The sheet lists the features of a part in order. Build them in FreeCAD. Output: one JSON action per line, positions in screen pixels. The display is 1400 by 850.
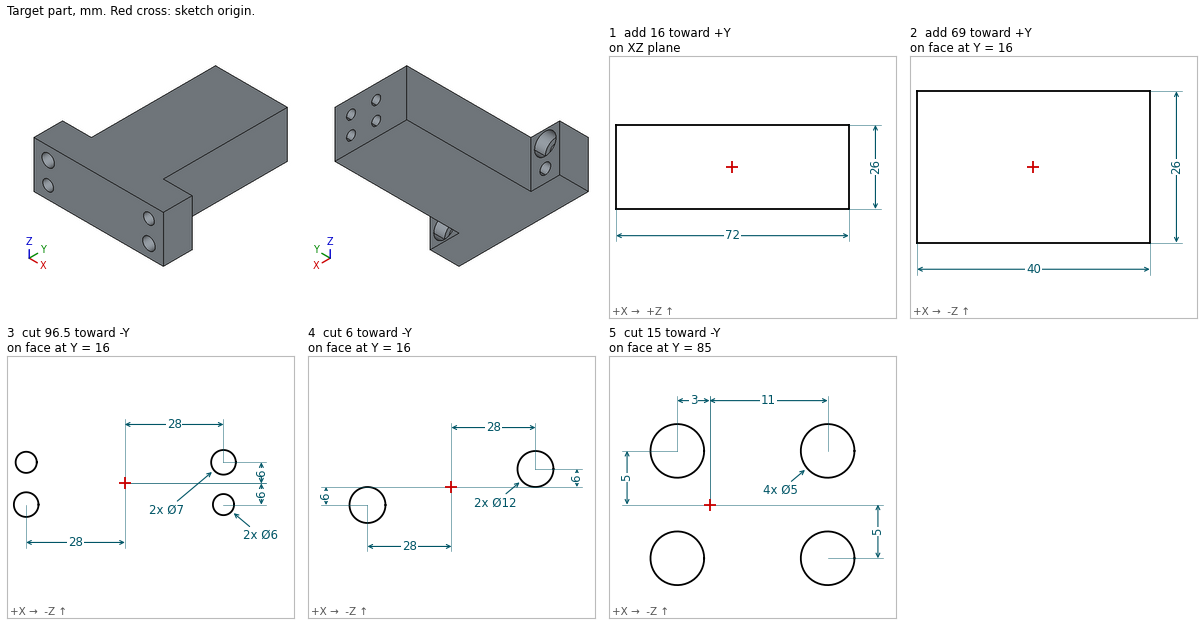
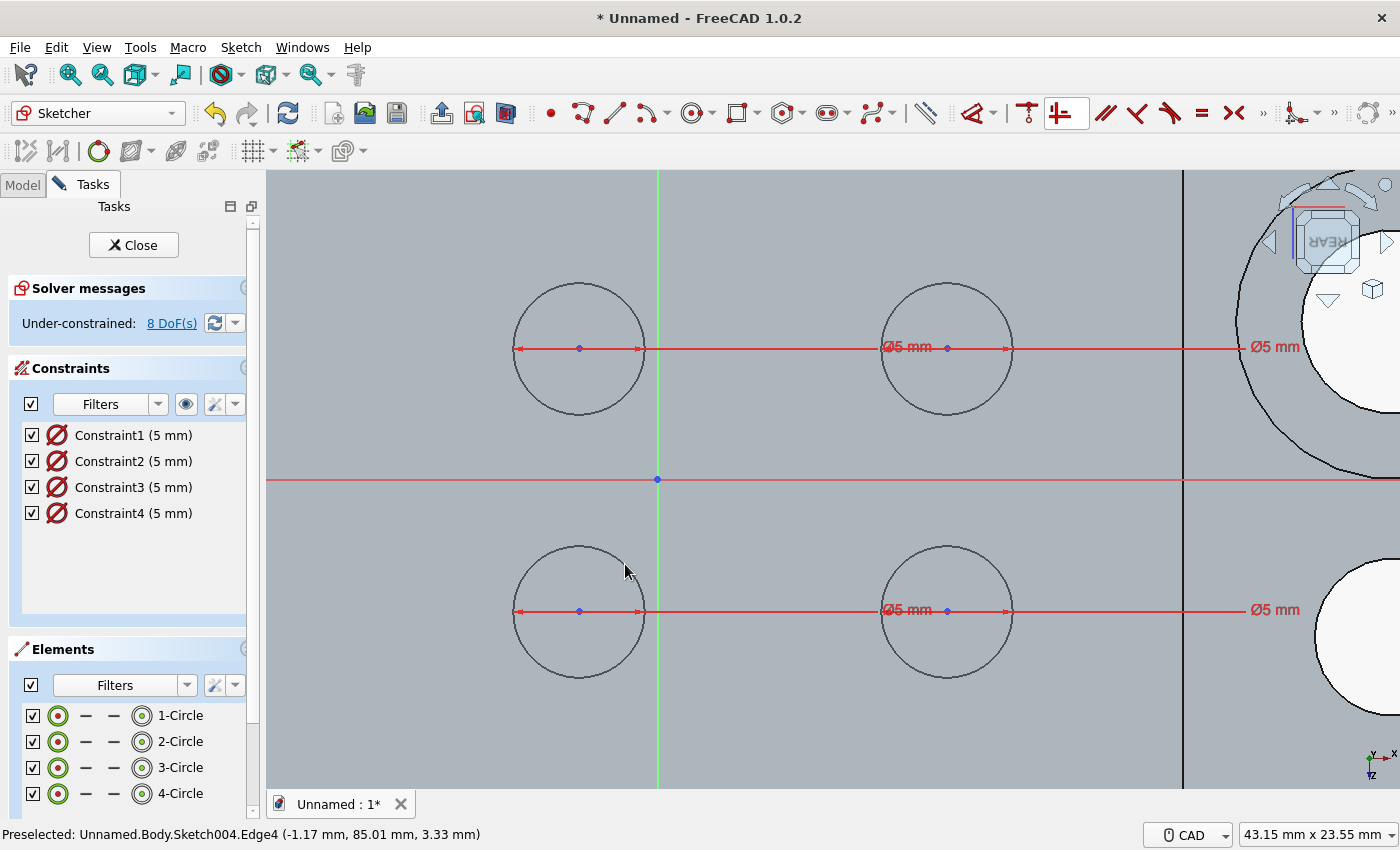
{"action": "left_click", "coordinate": [579, 349]}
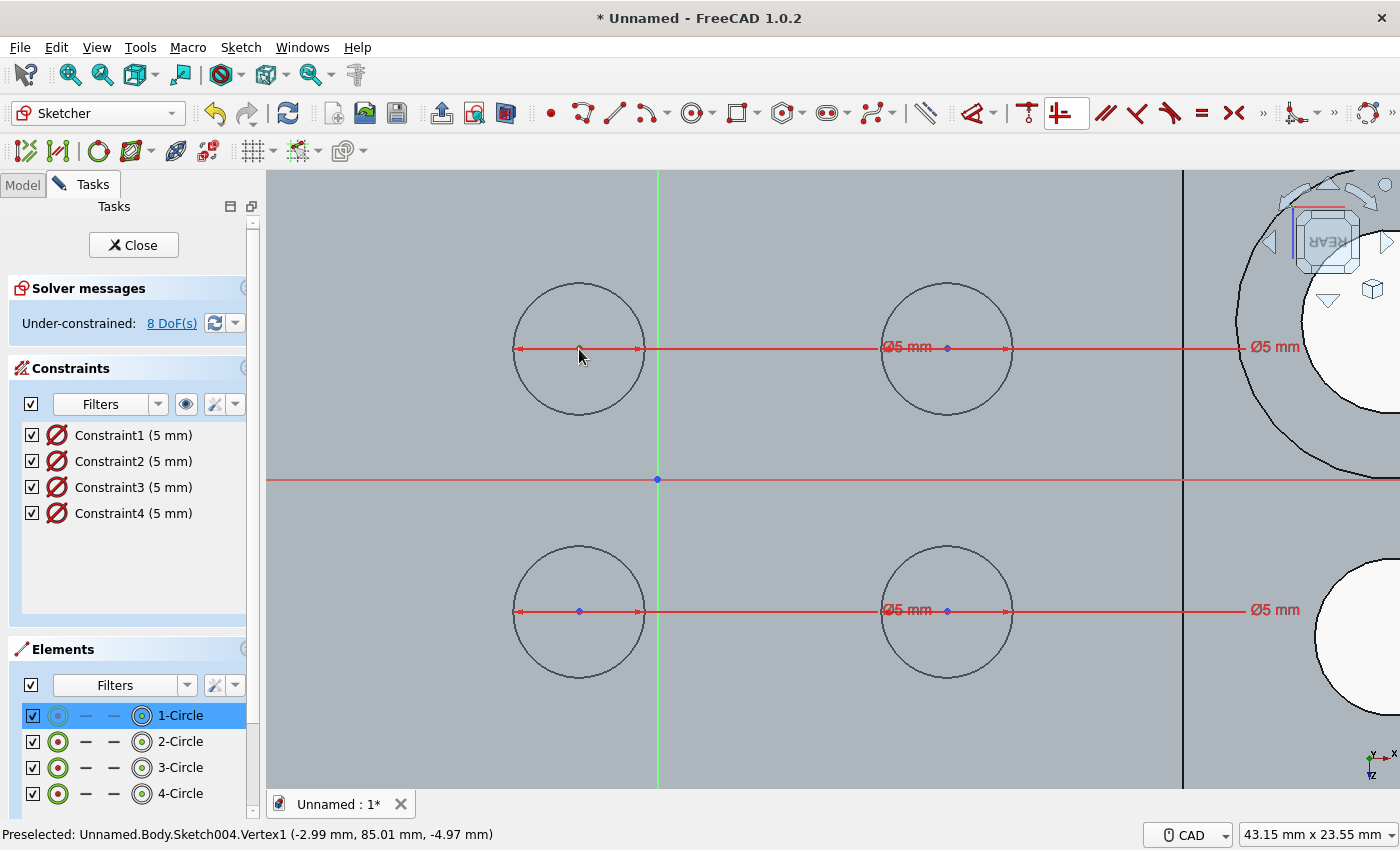
{"action": "left_click", "coordinate": [947, 349]}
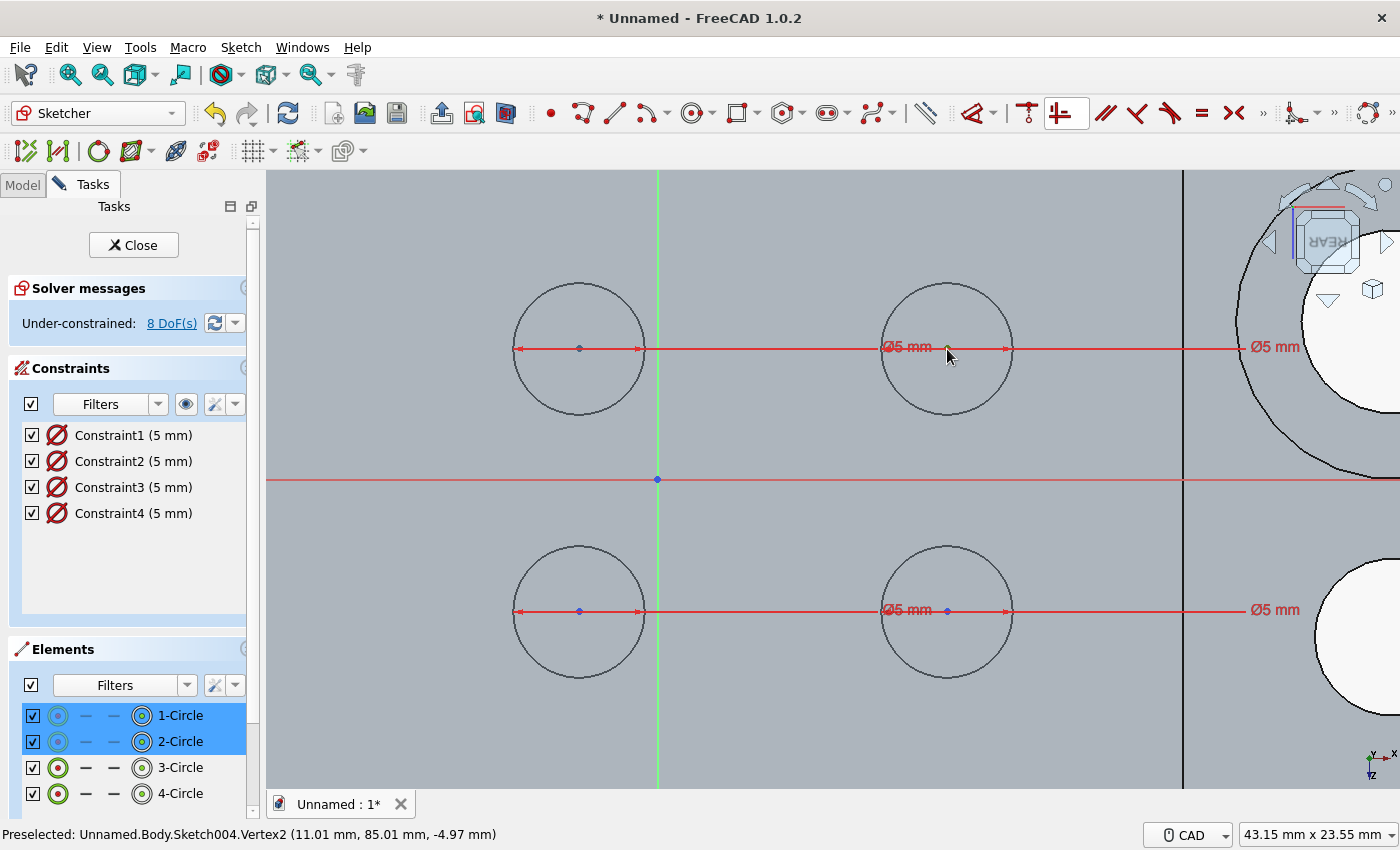
{"action": "key", "text": "h"}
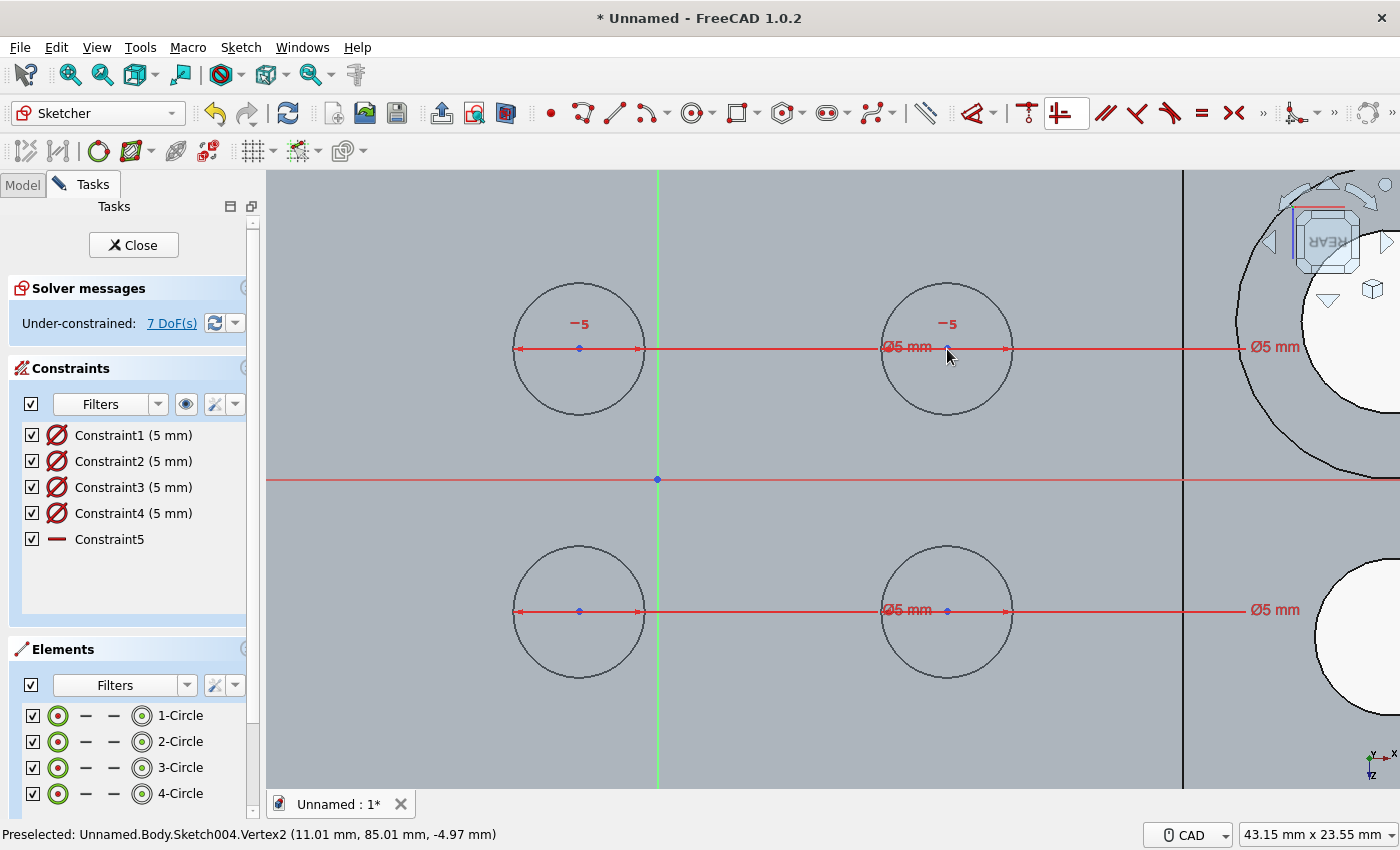
{"action": "left_click", "coordinate": [947, 349]}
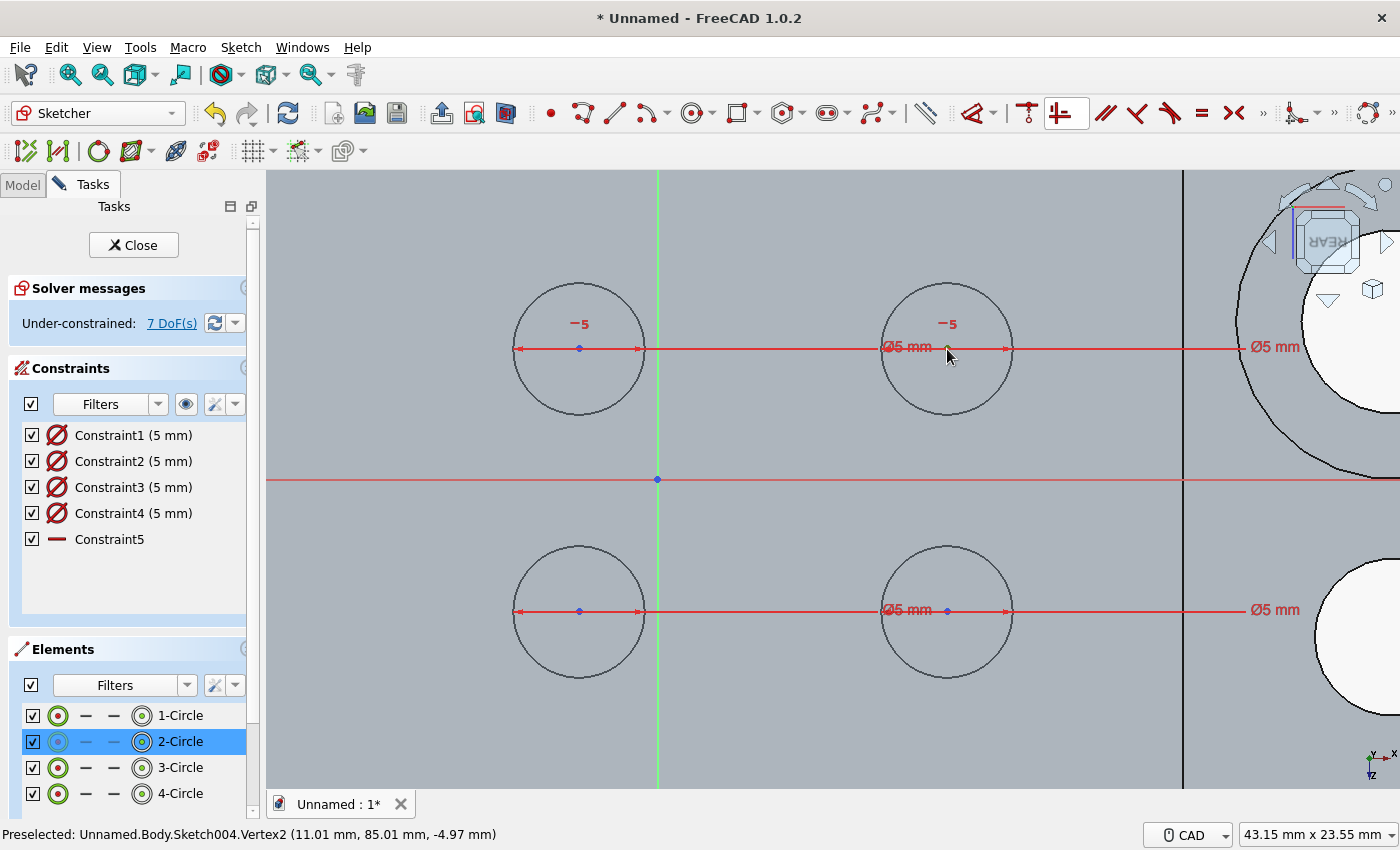
{"action": "left_click", "coordinate": [947, 612]}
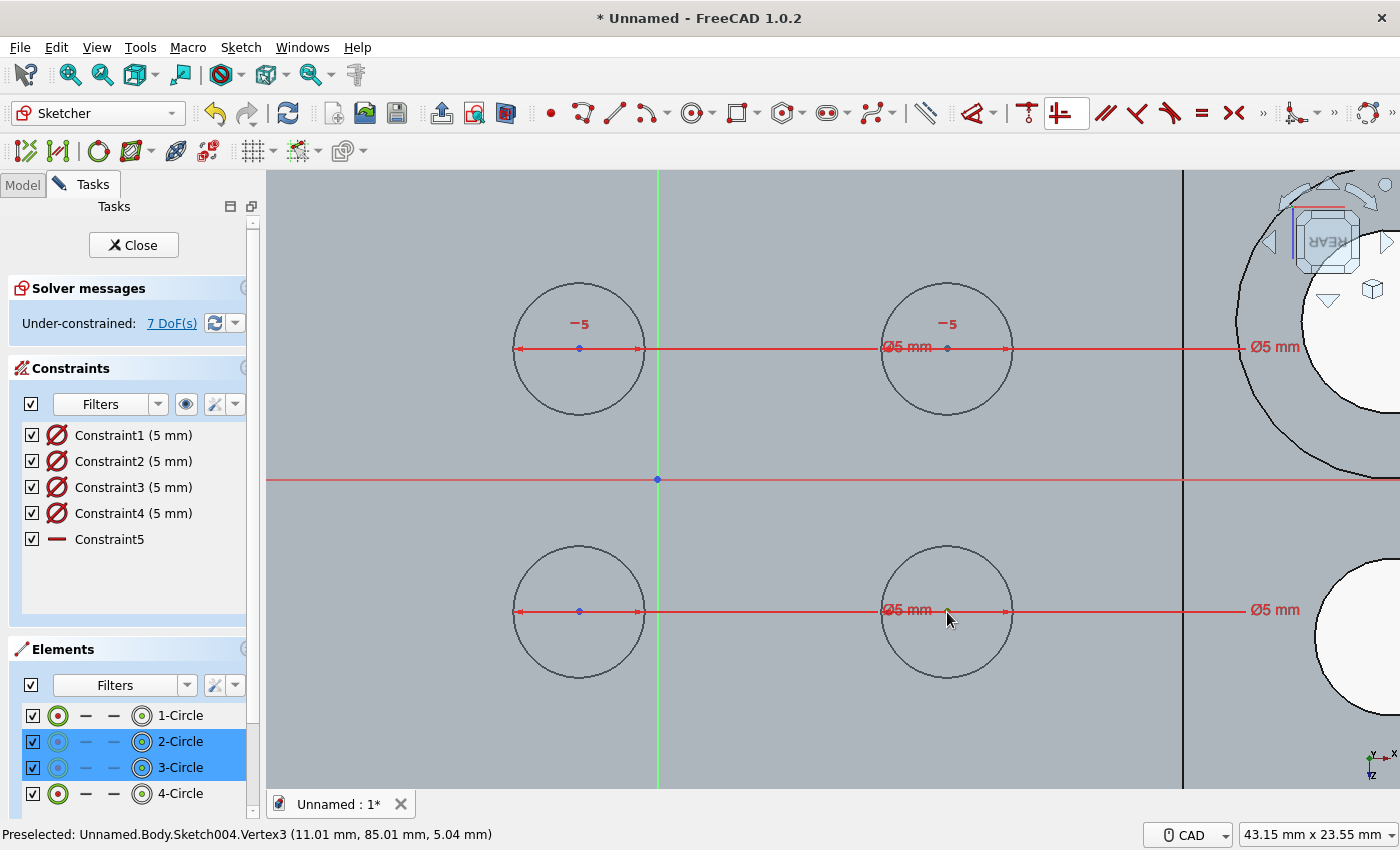
{"action": "key", "text": "v"}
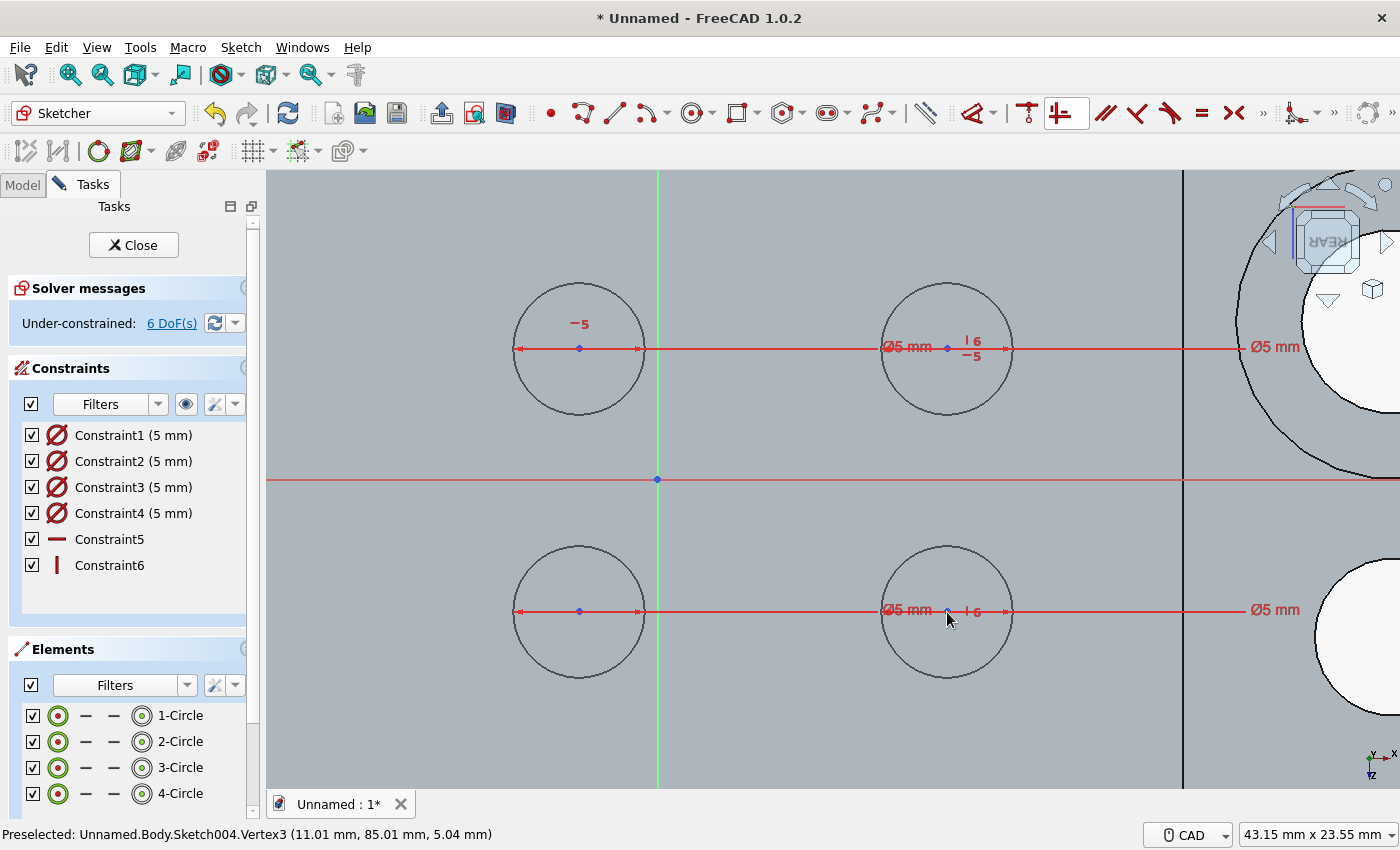
{"action": "left_click", "coordinate": [579, 349]}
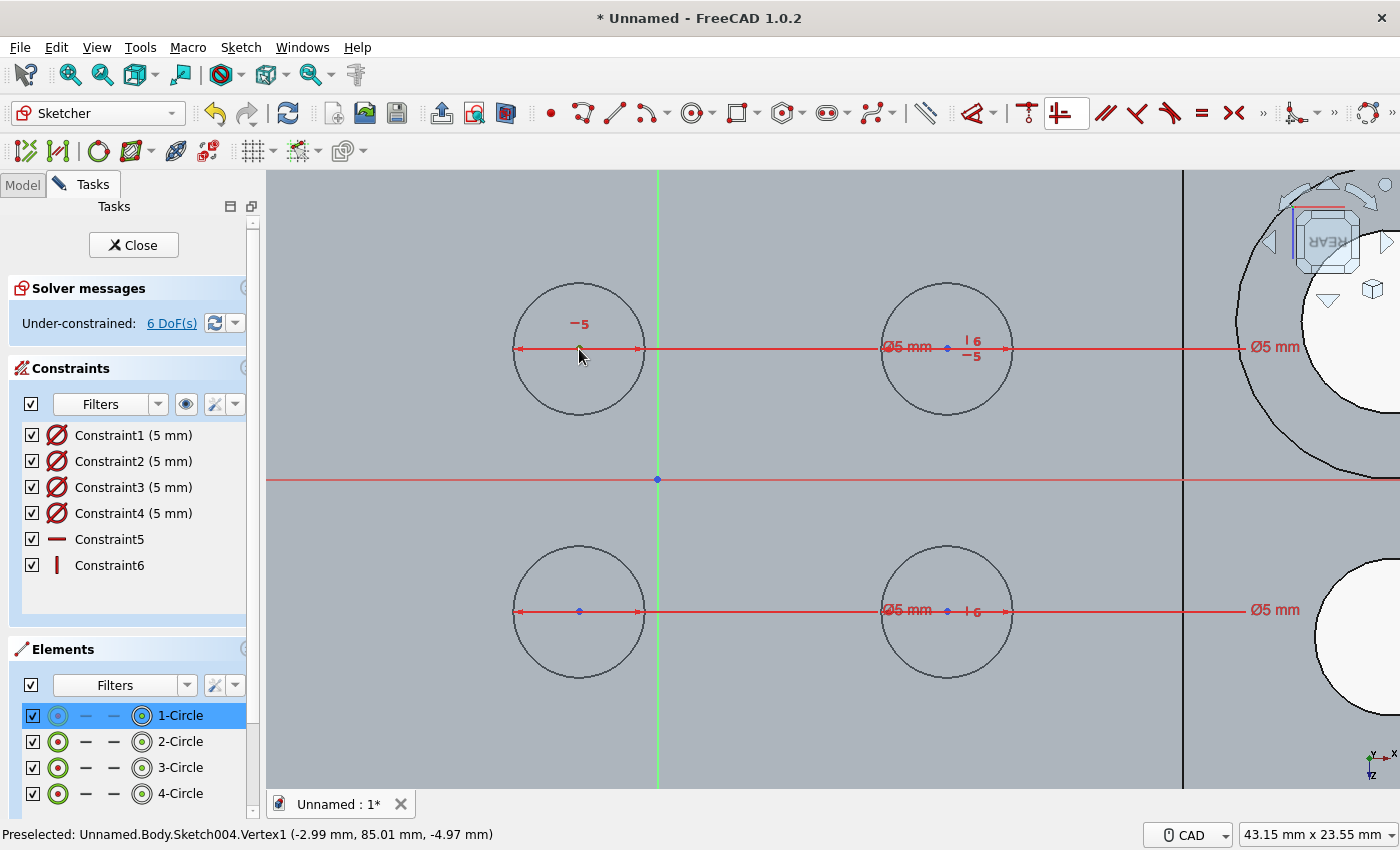
{"action": "left_click", "coordinate": [579, 612]}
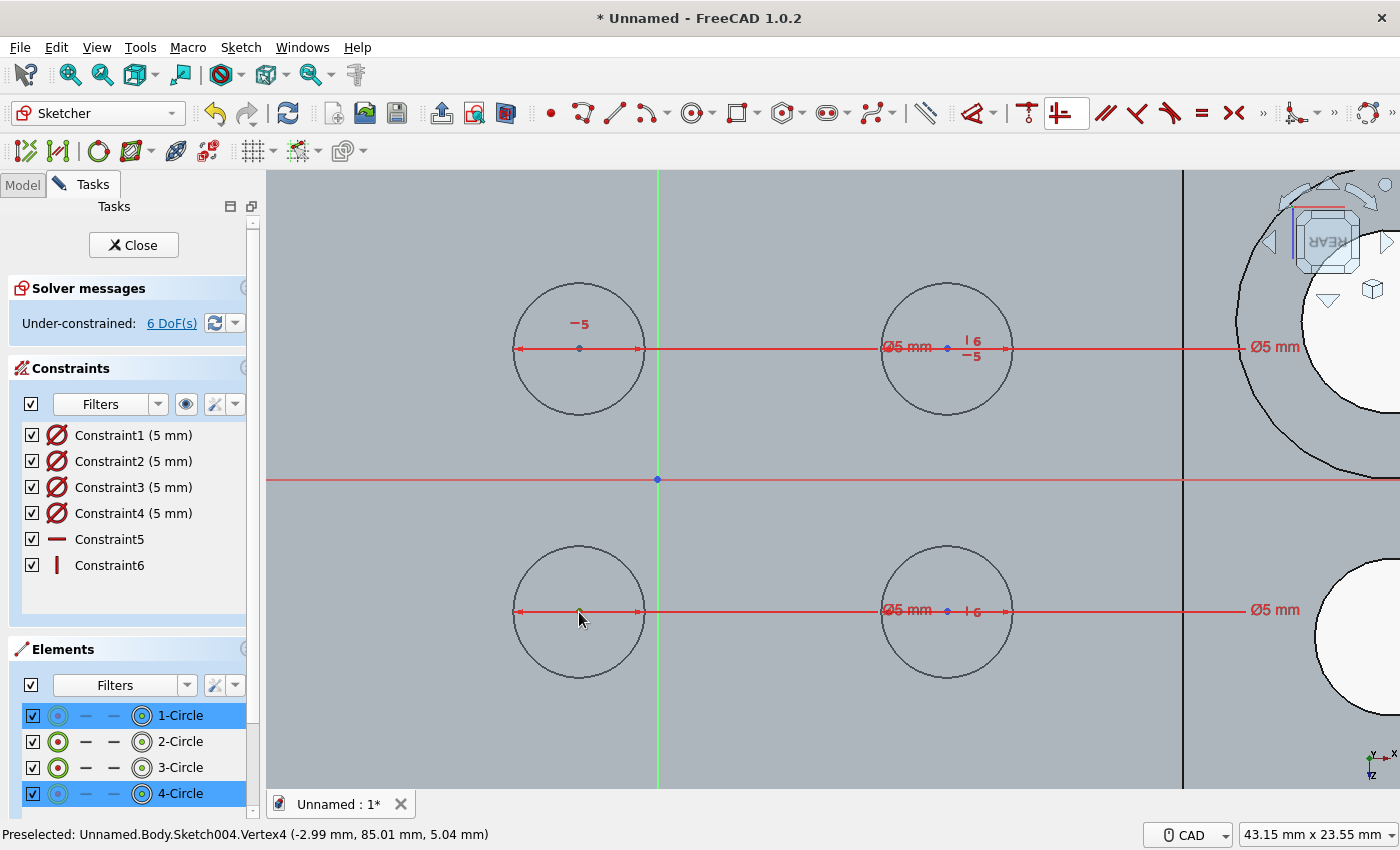
{"action": "key", "text": "v"}